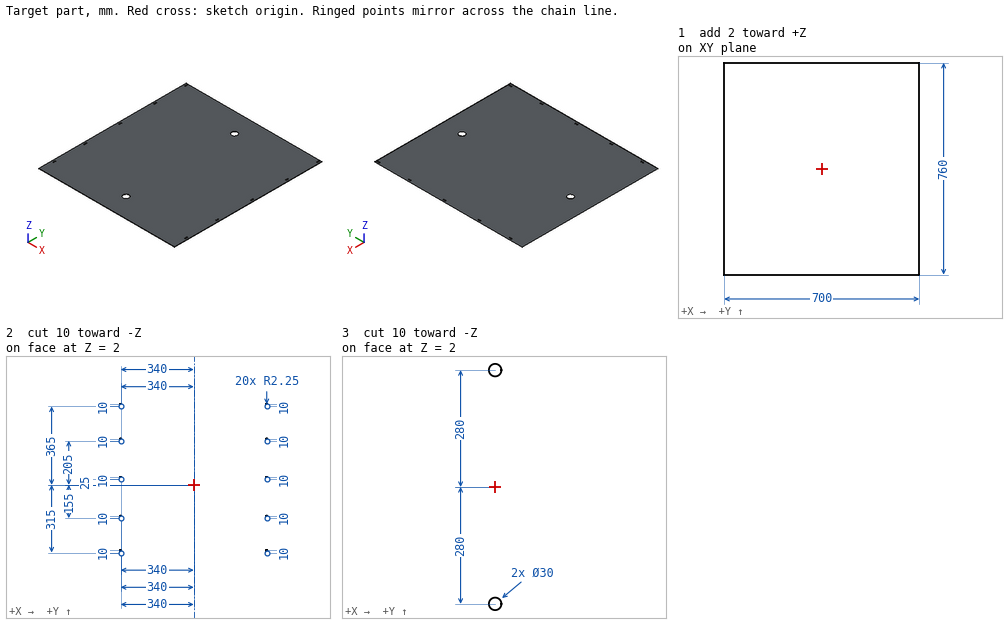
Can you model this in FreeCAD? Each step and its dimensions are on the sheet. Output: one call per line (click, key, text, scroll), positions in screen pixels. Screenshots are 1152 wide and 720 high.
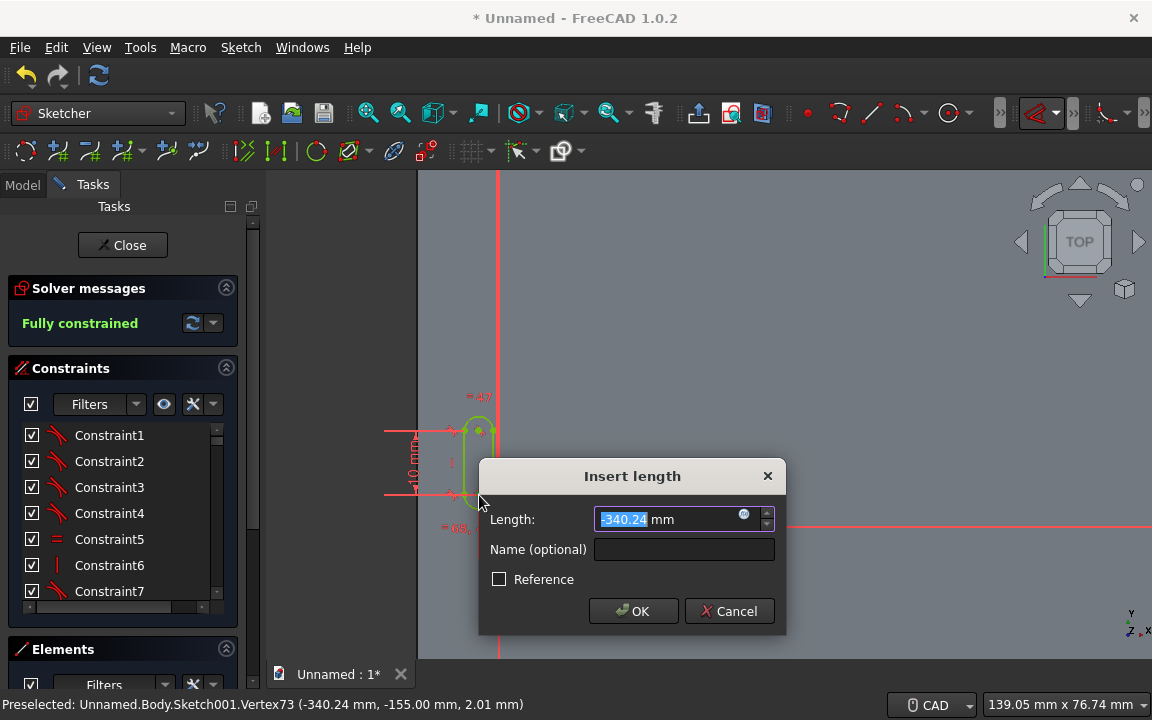
text(-340)
key(Return)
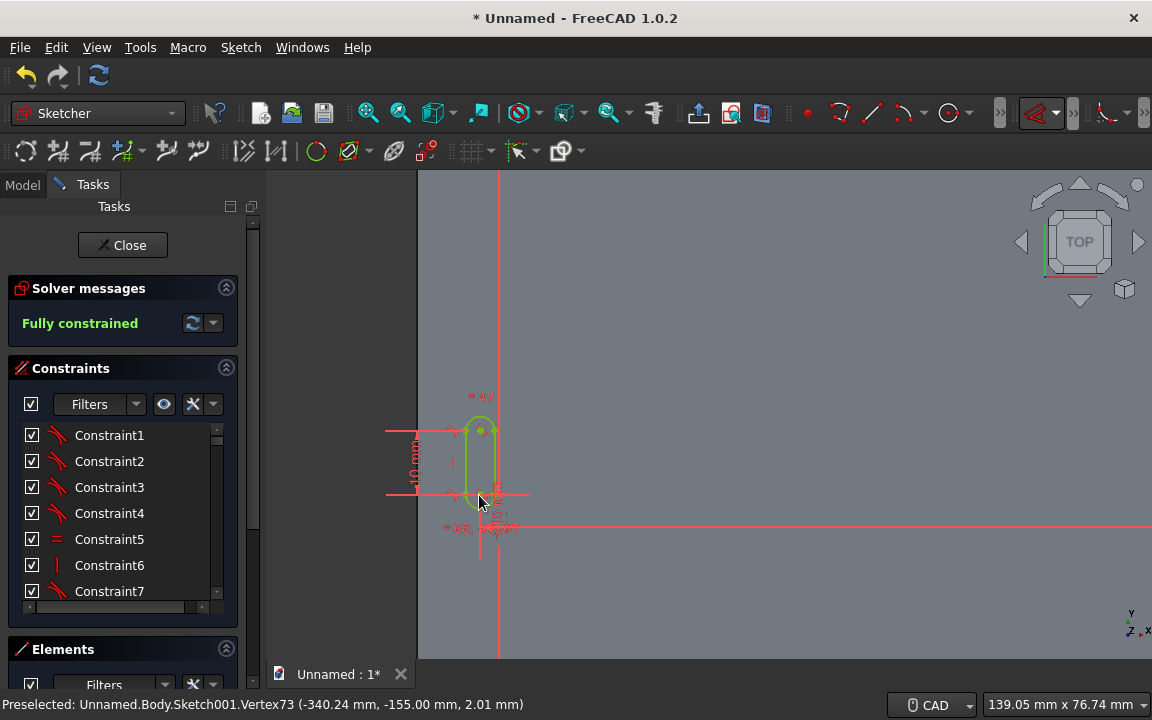
click(123, 245)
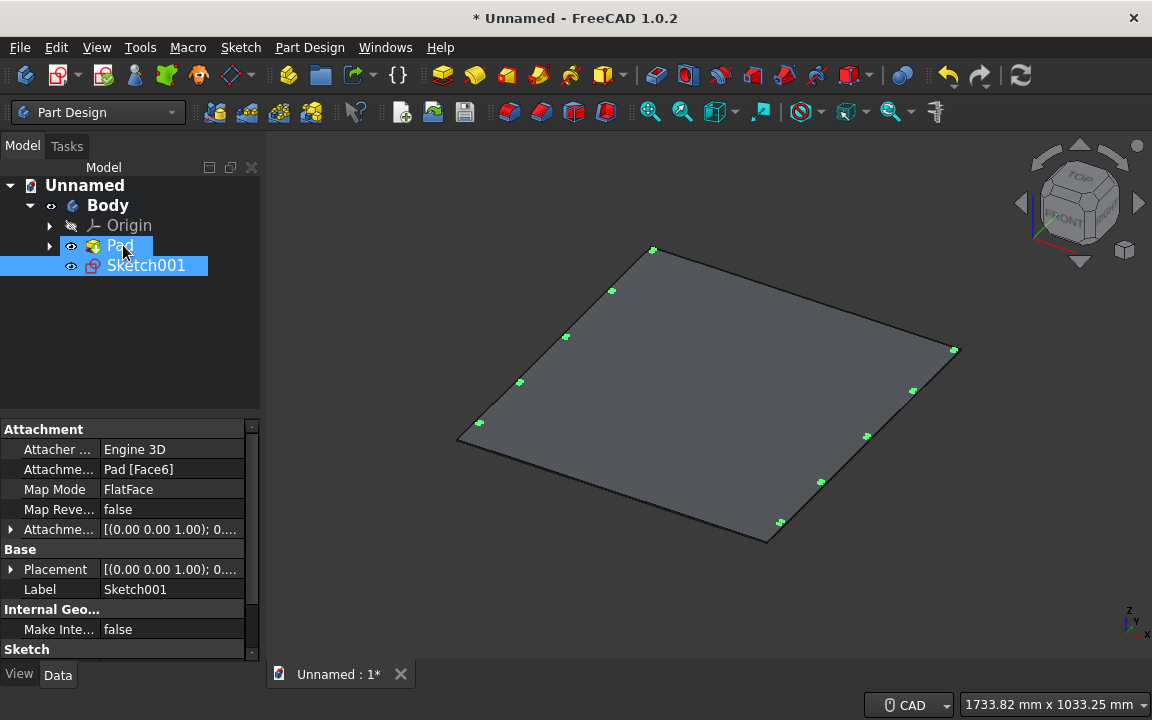
click(658, 76)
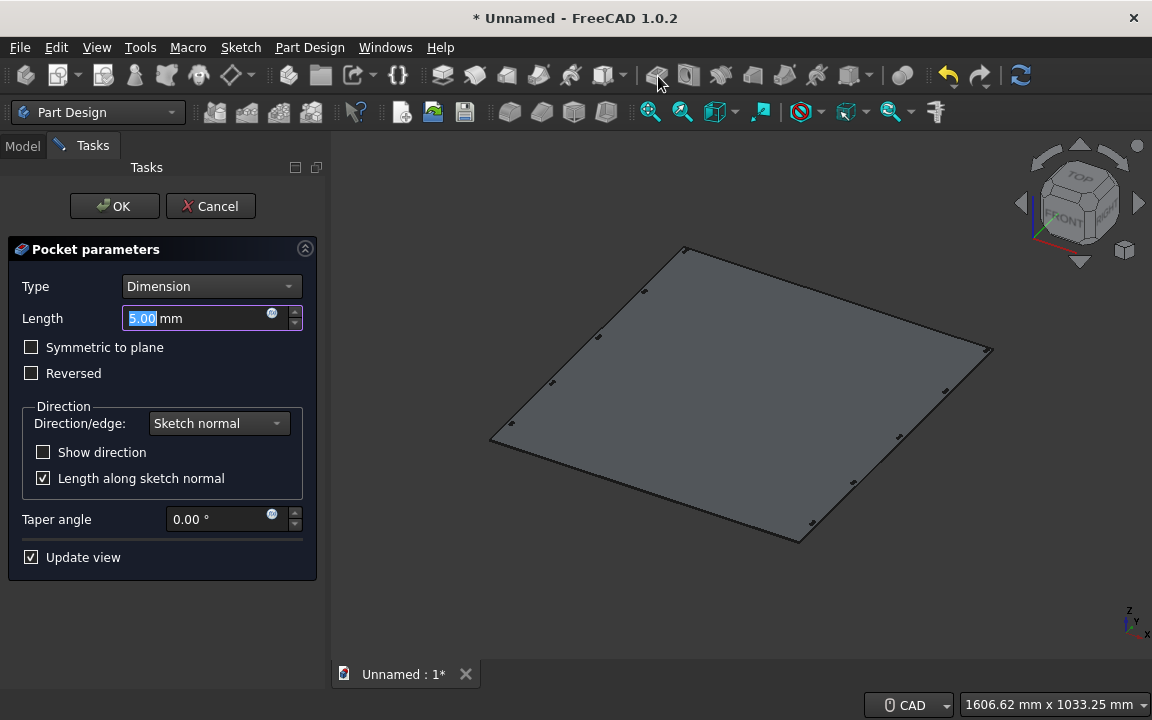
text(10)
key(Tab)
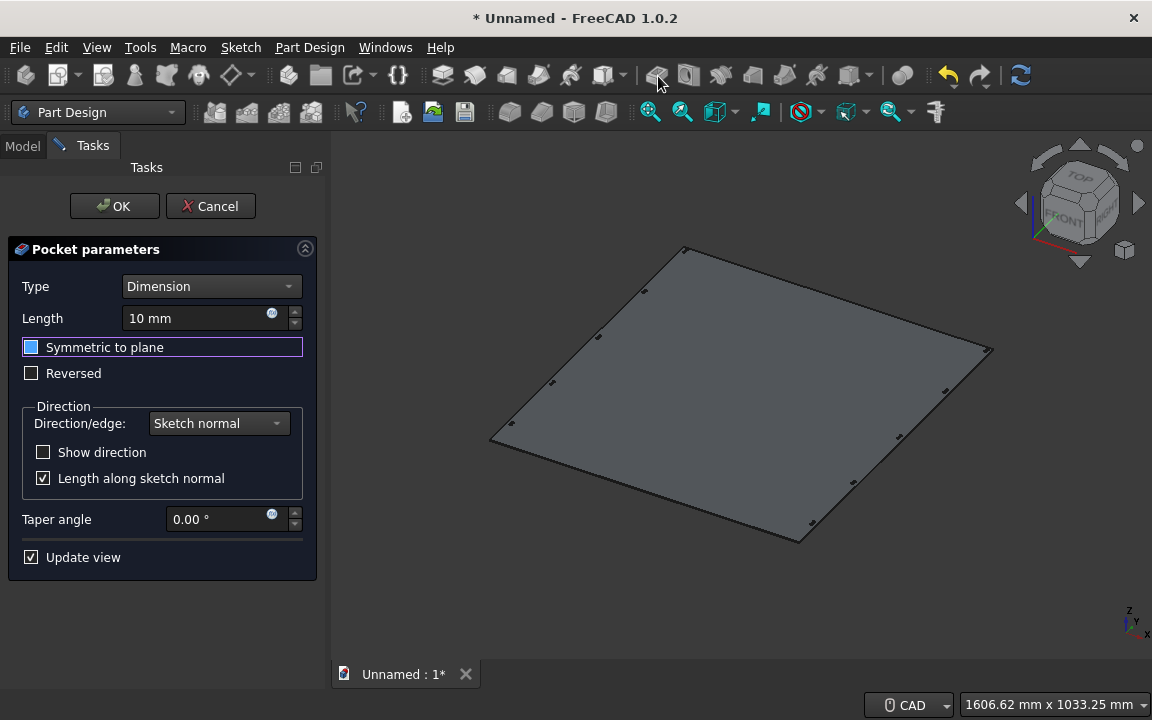
click(115, 206)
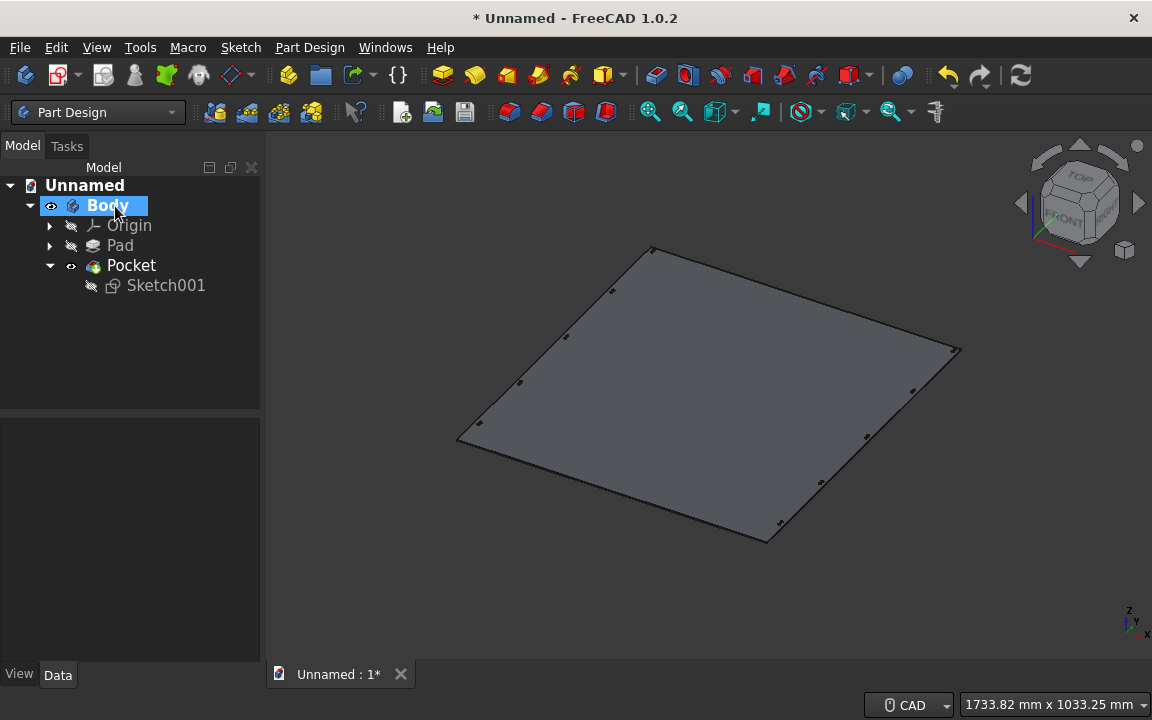
click(709, 394)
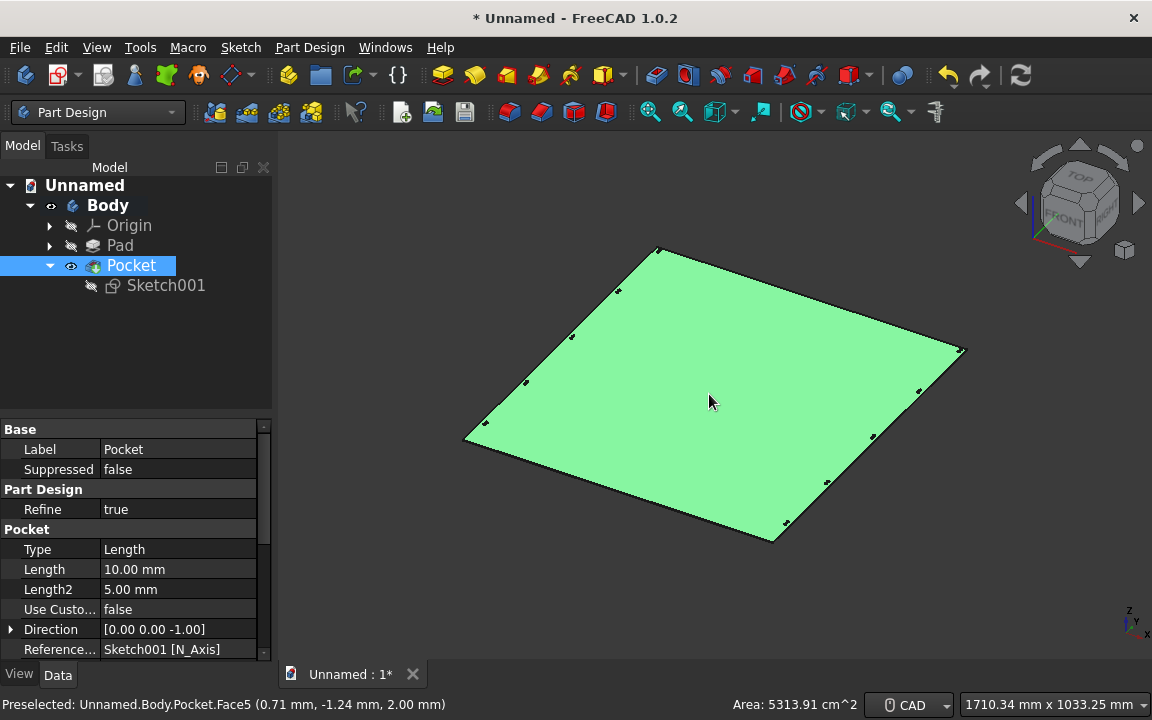
click(58, 76)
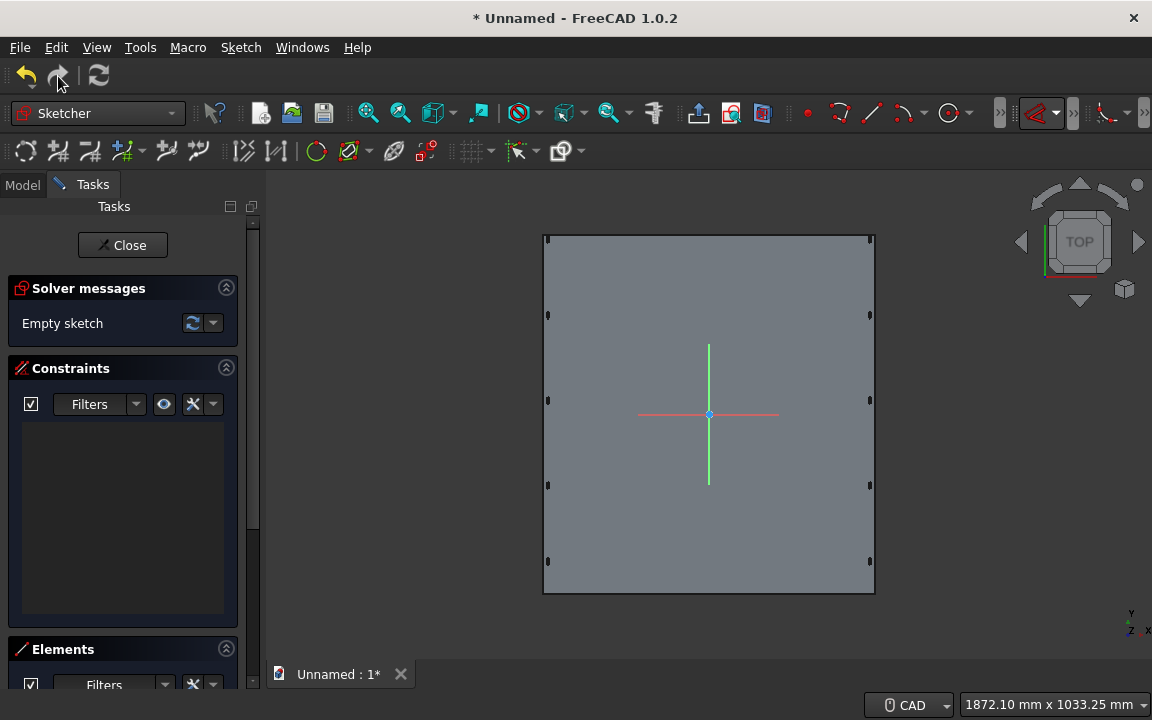
click(950, 114)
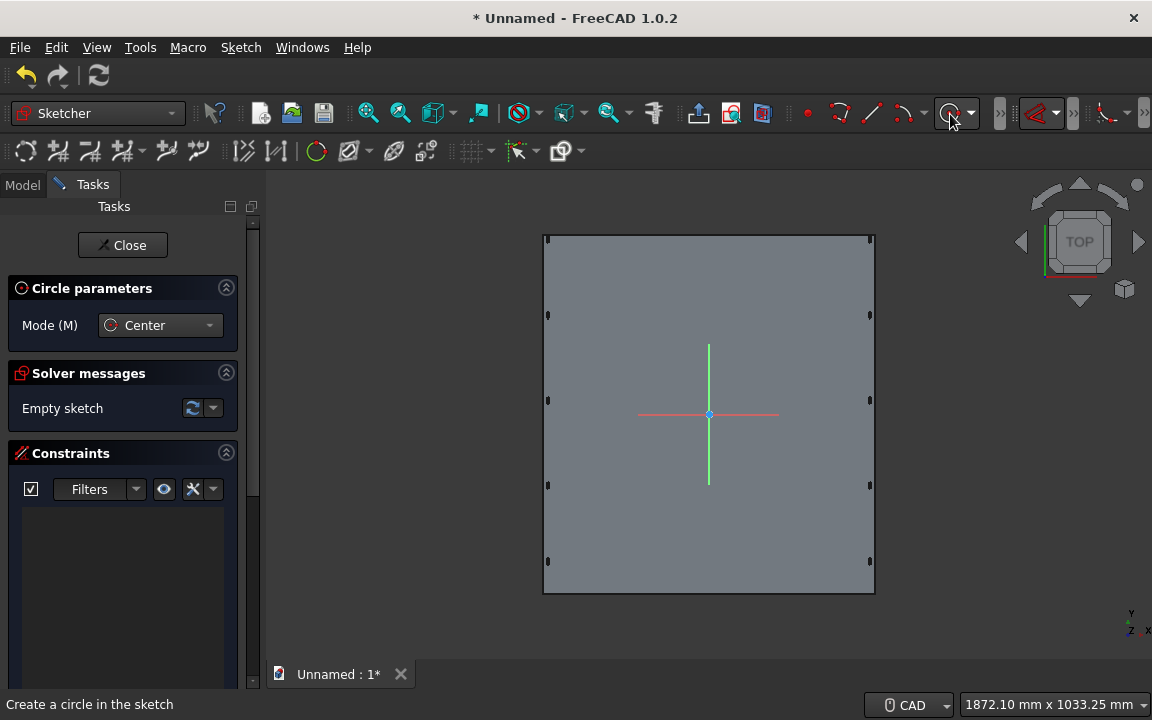
scroll(709, 547, up, 6)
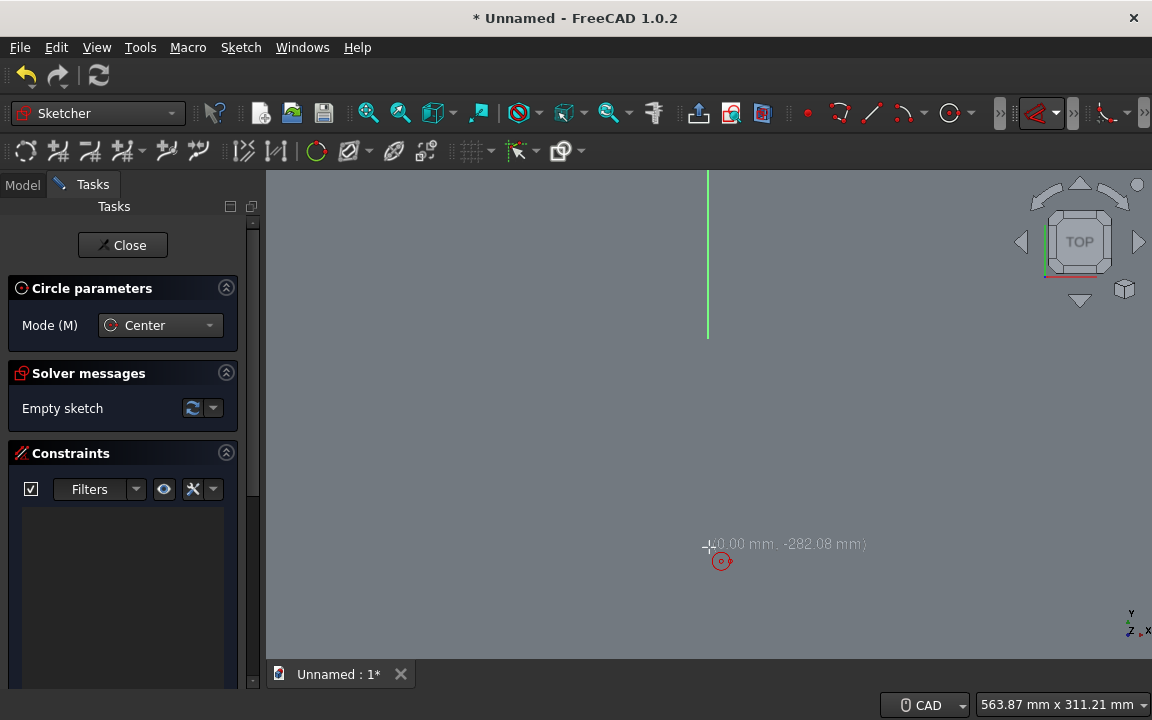
click(708, 545)
move(725, 529)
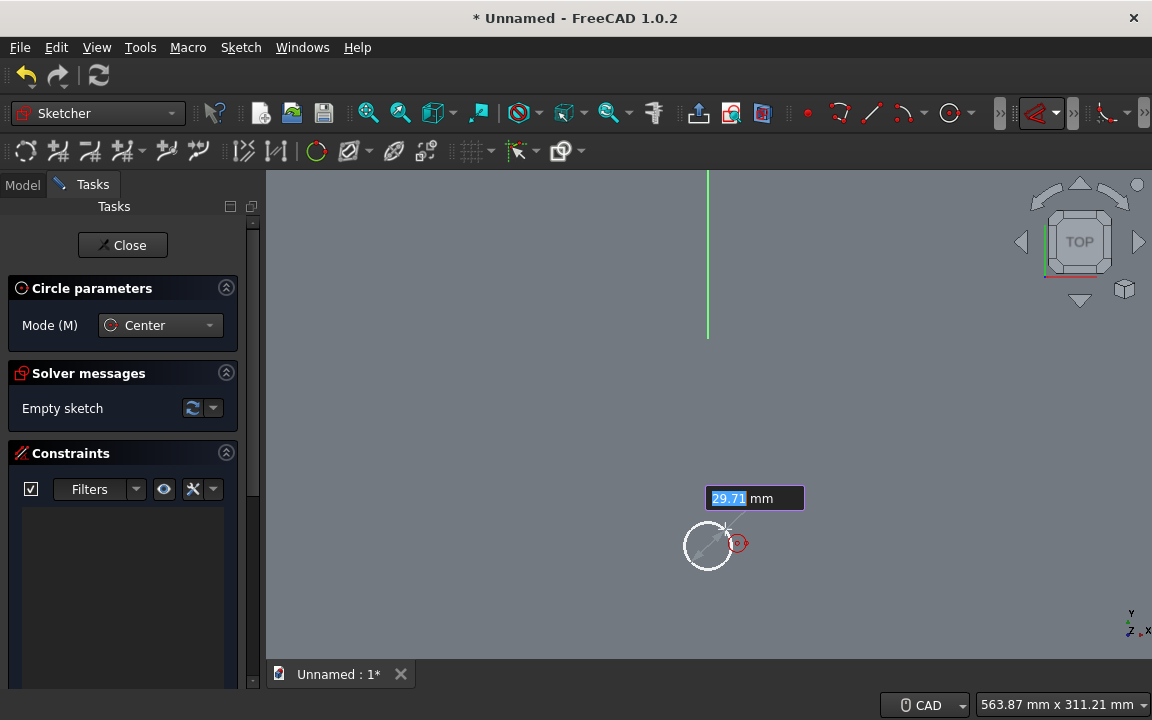
text(30)
key(Return)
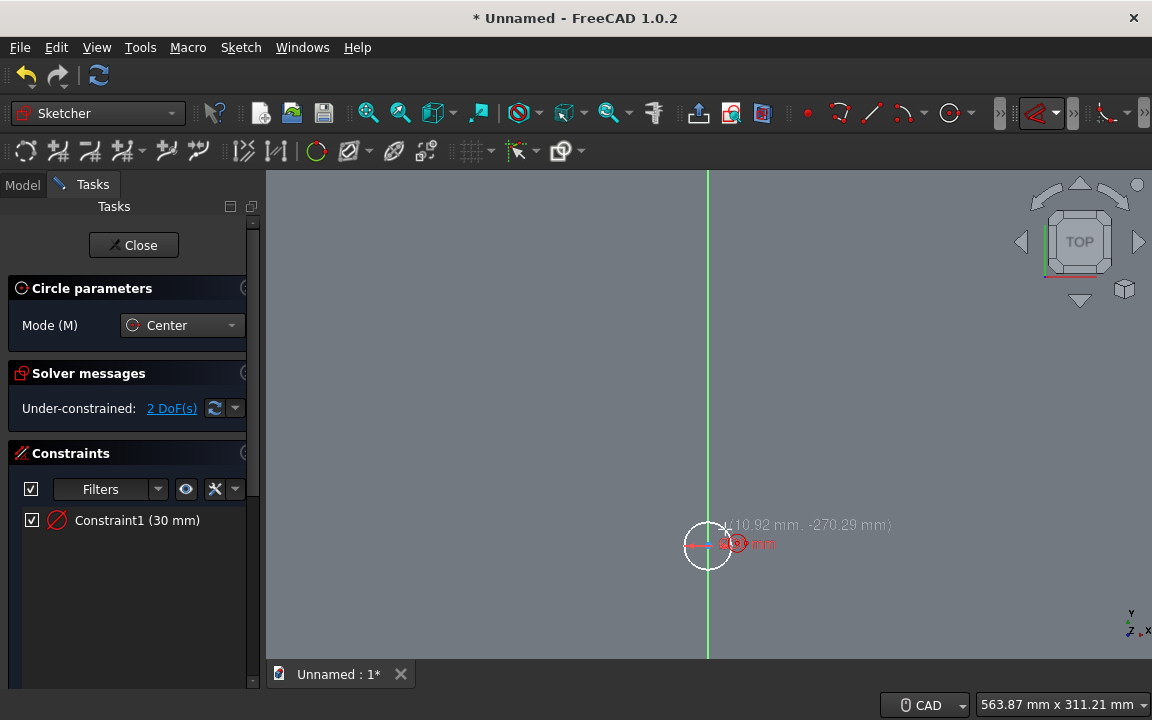
scroll(611, 548, down, 6)